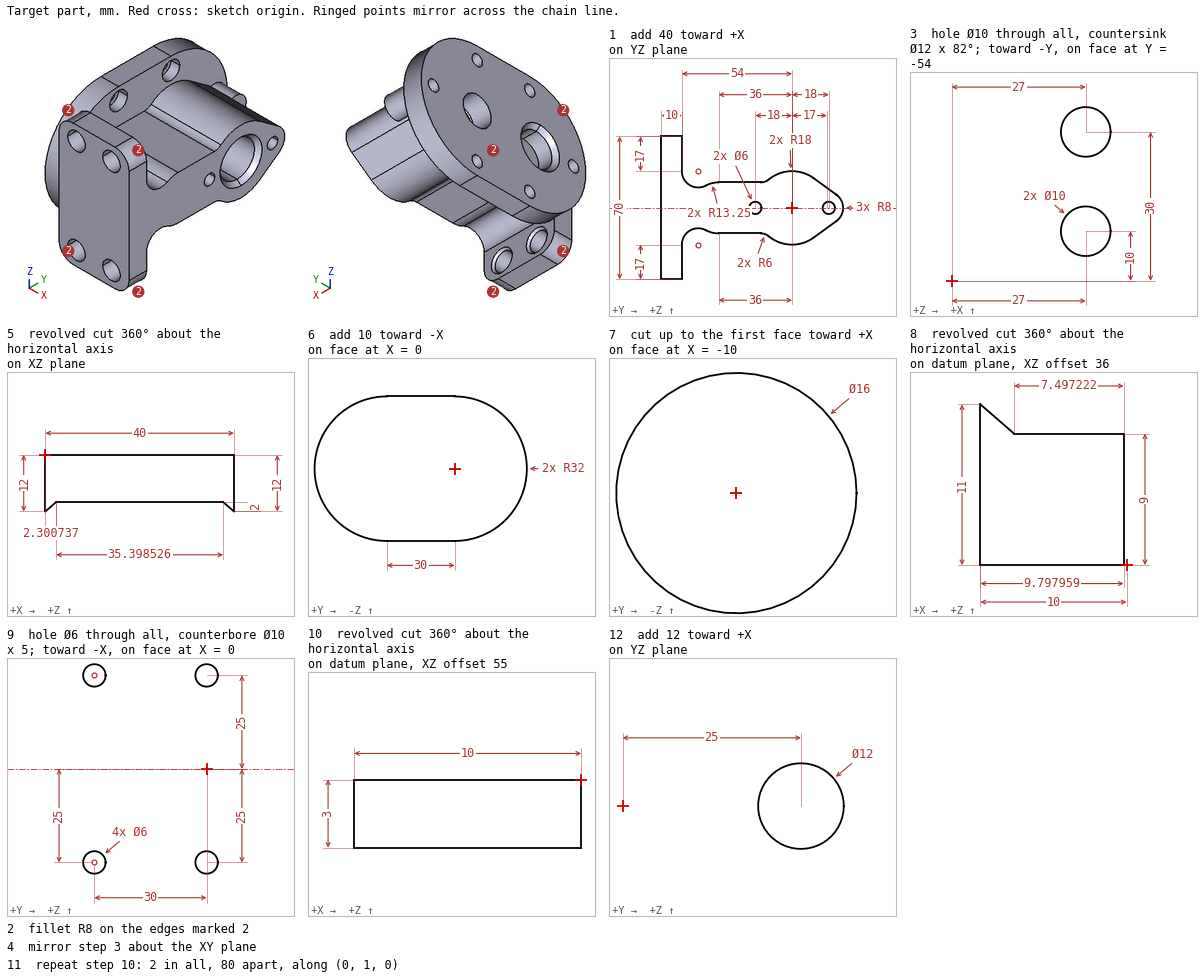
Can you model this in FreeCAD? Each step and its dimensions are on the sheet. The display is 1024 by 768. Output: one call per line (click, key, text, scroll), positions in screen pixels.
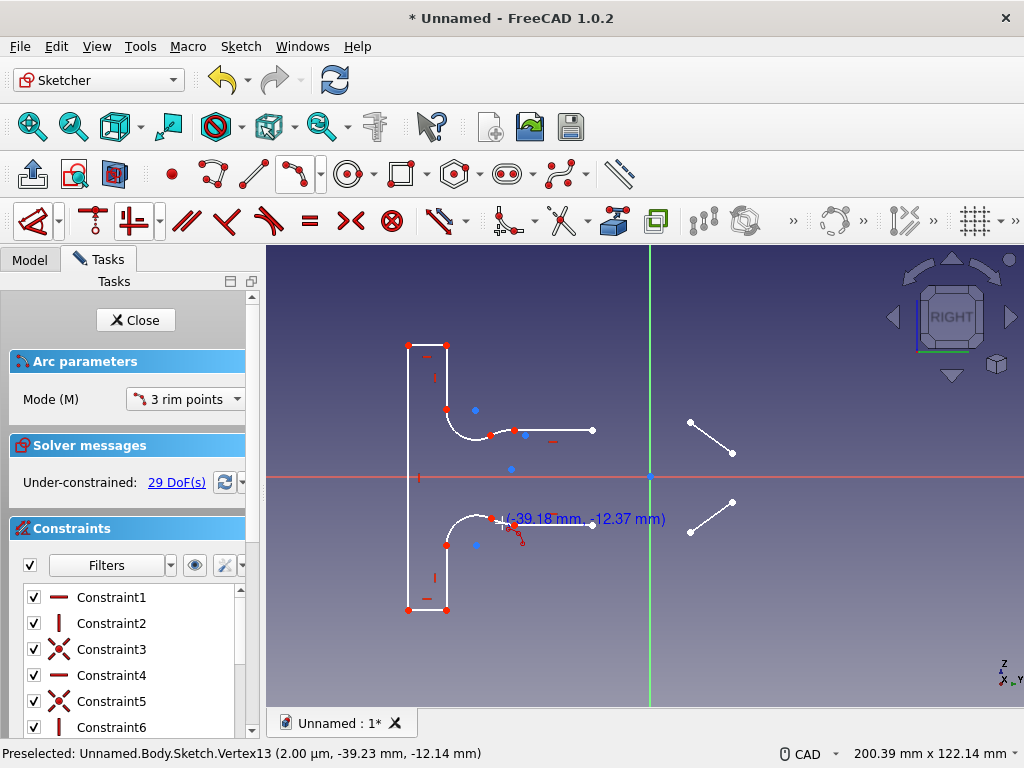
click(592, 525)
click(607, 529)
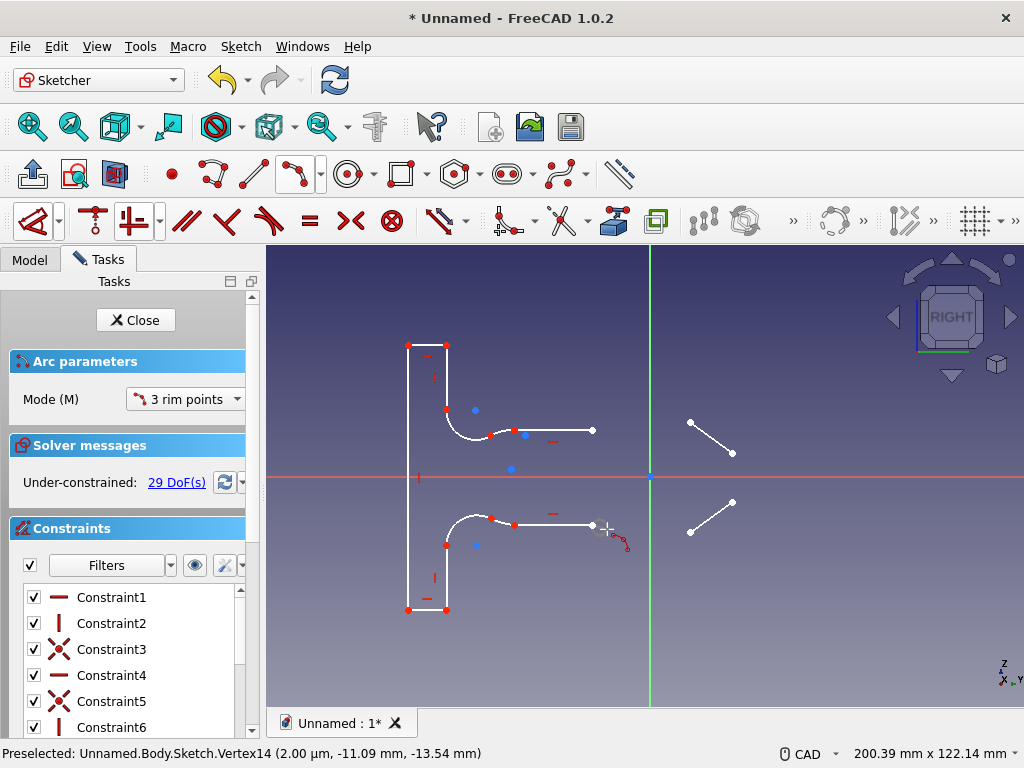
scroll(600, 525, up, 13)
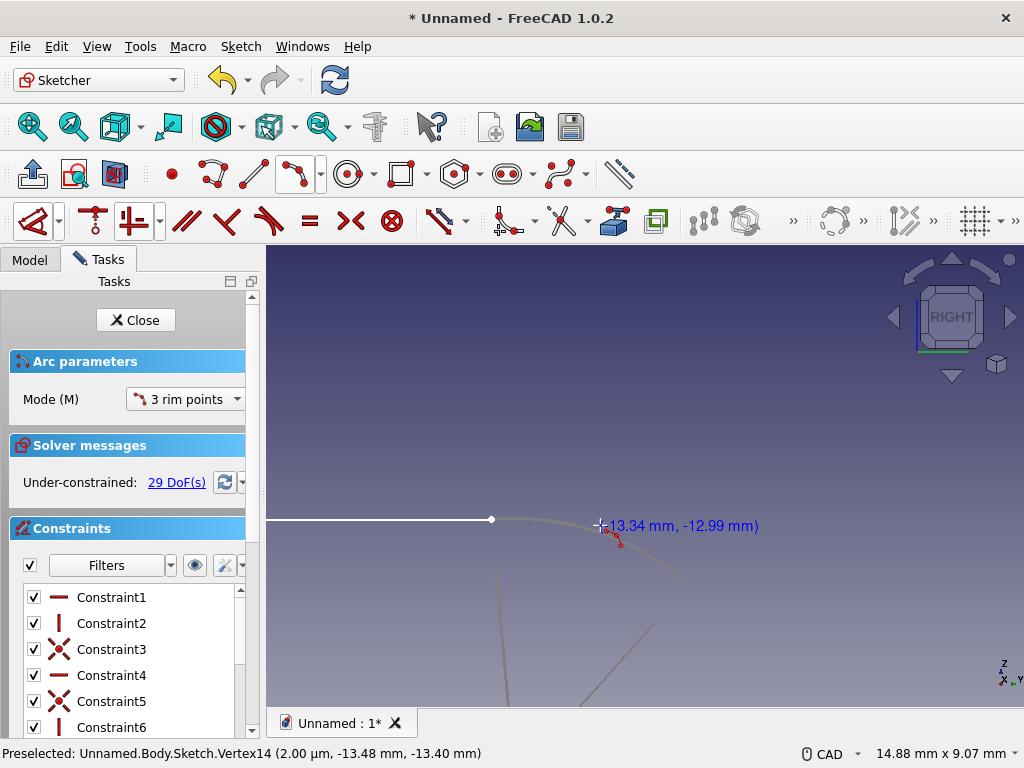
click(599, 524)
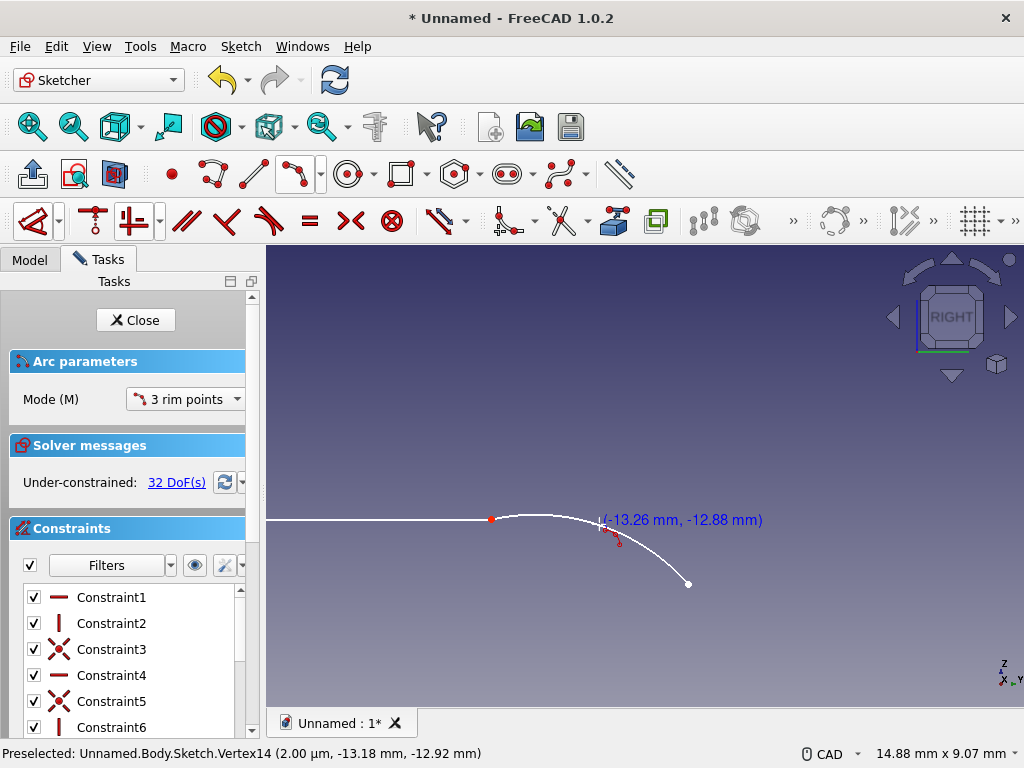
scroll(600, 525, down, 13)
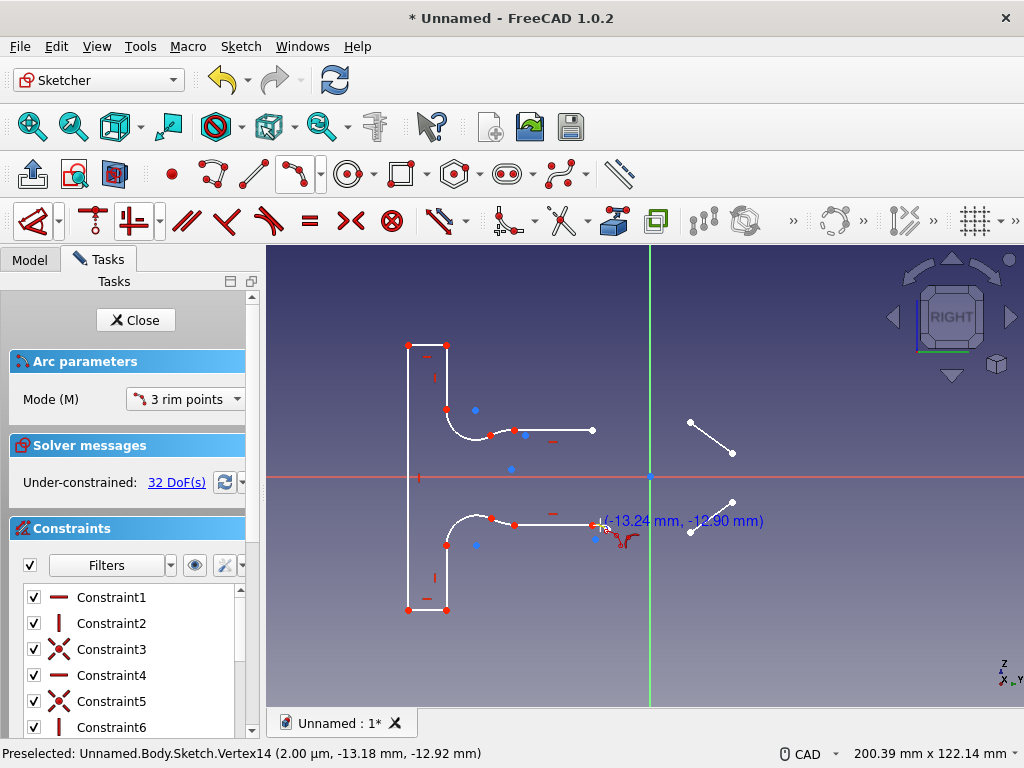
click(607, 530)
click(691, 533)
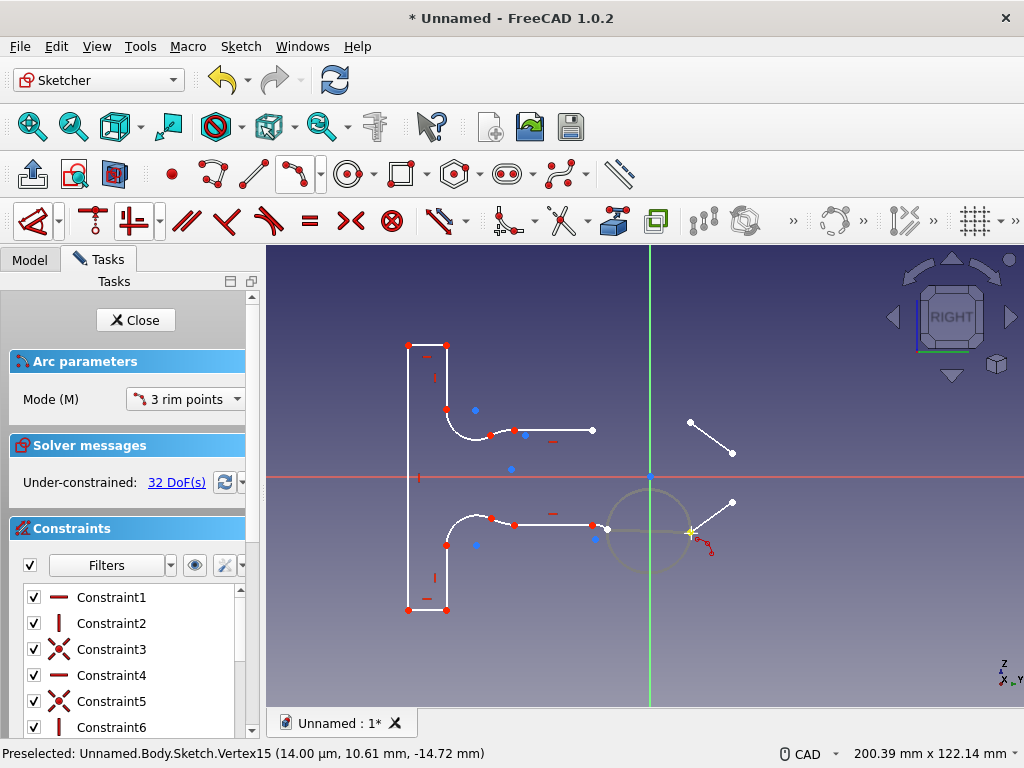
scroll(631, 542, up, 2)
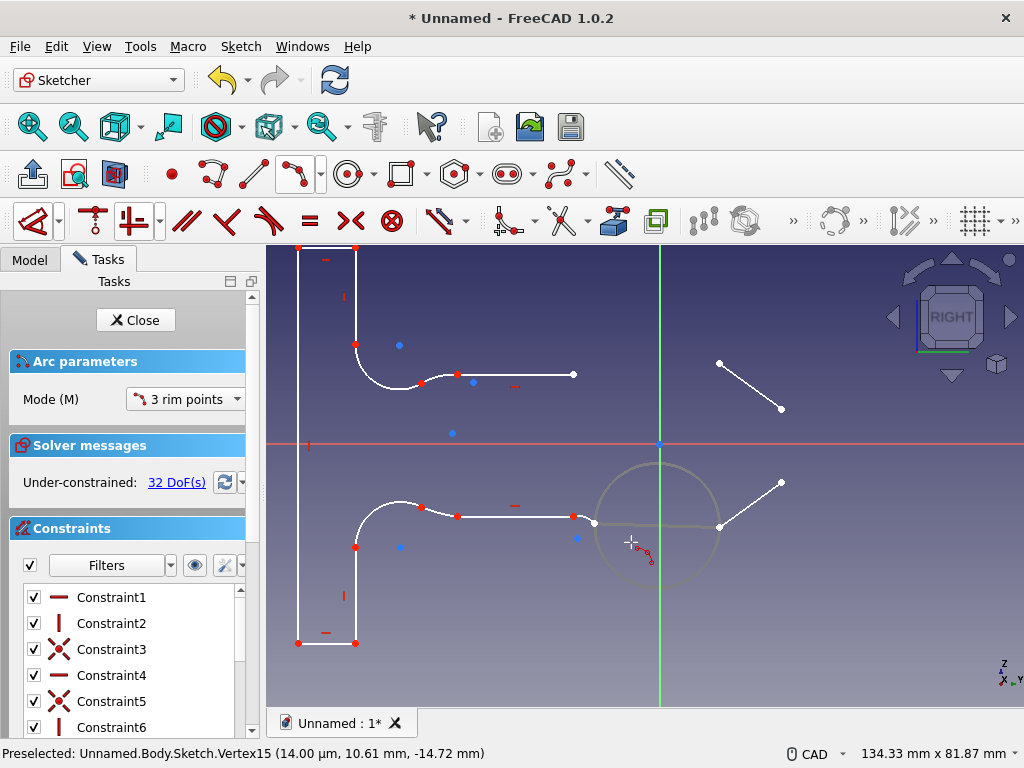
click(630, 542)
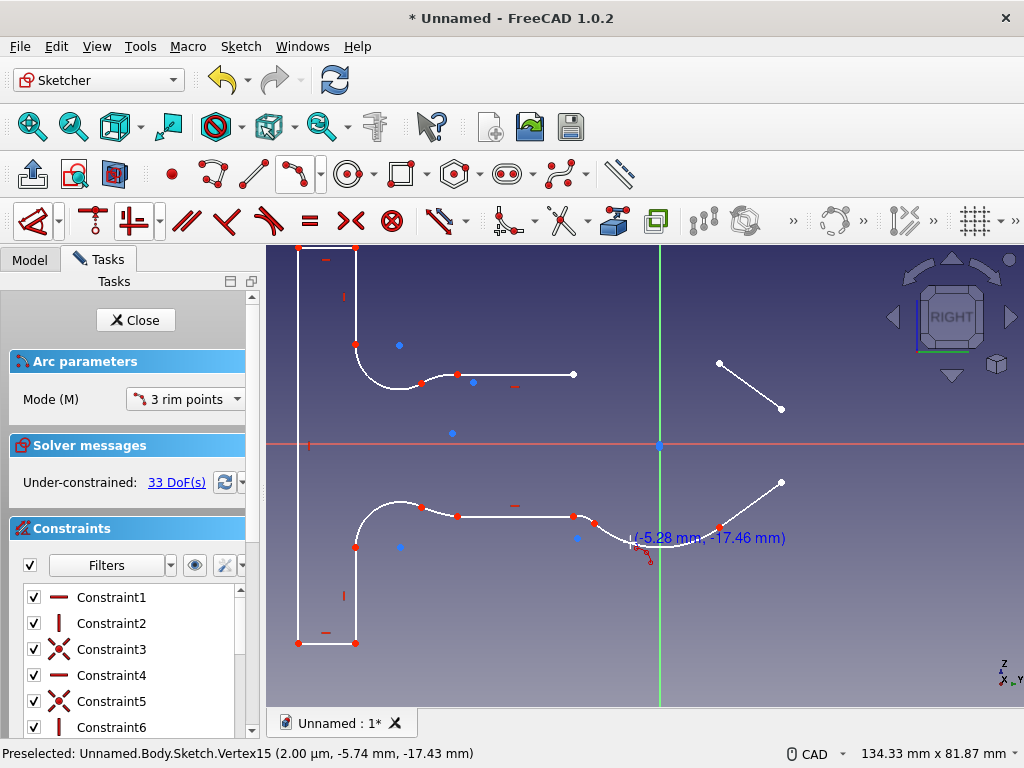
click(782, 482)
click(782, 409)
click(798, 461)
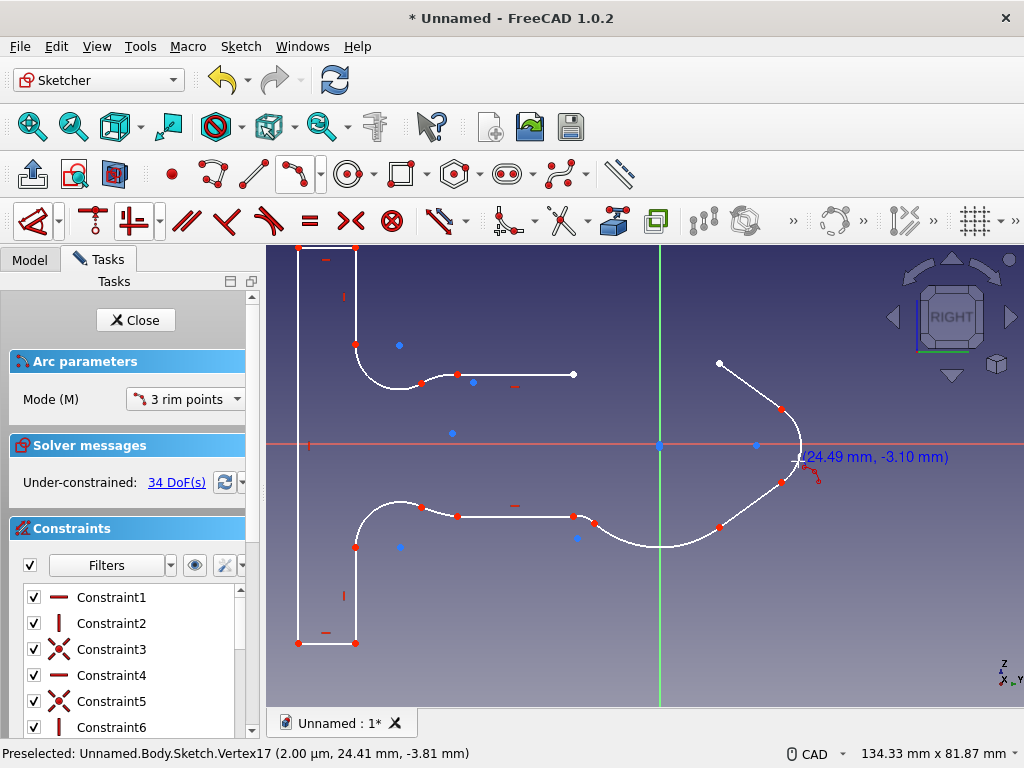
click(720, 364)
click(595, 366)
click(683, 346)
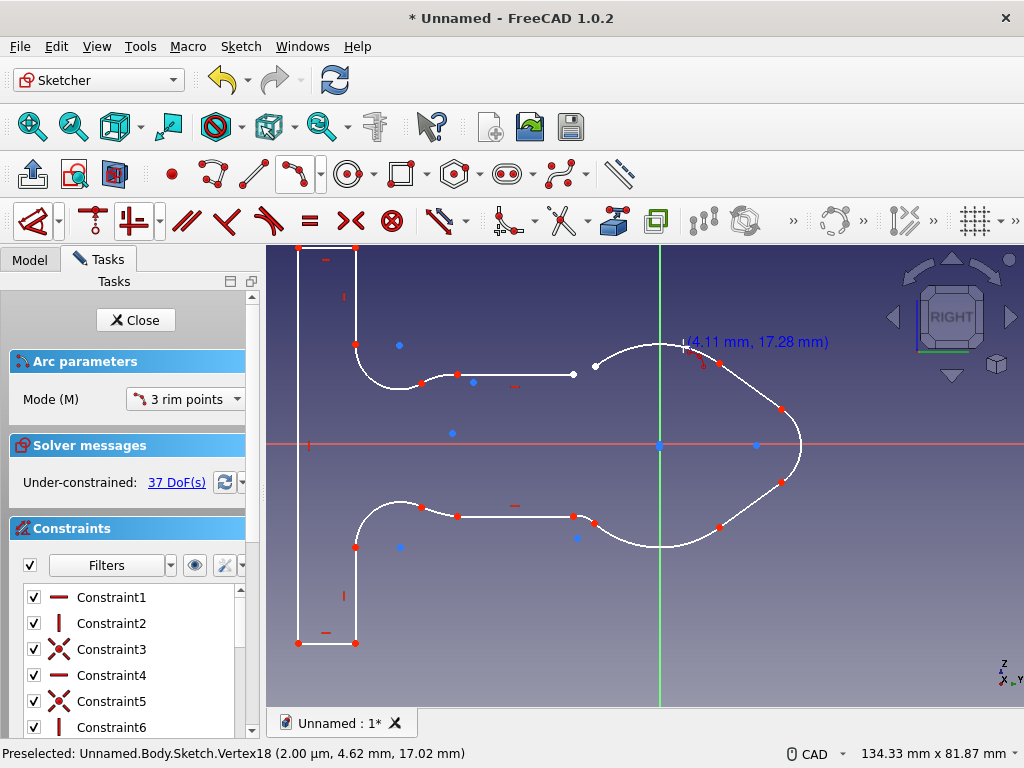
click(595, 367)
click(573, 375)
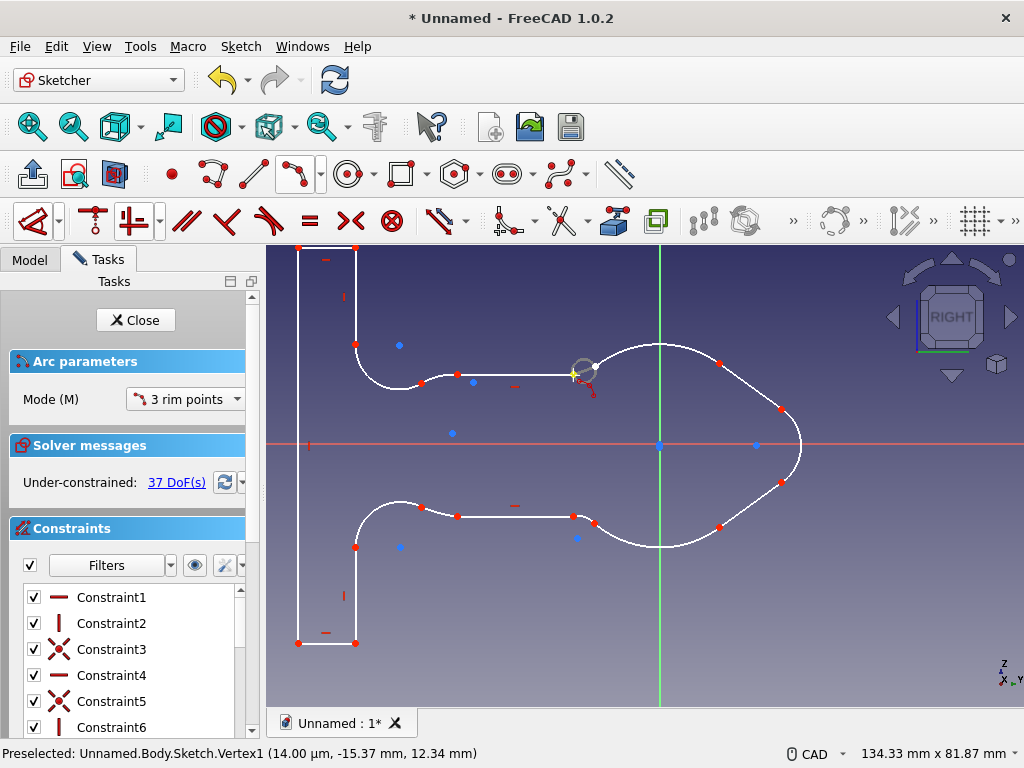
scroll(585, 372, up, 11)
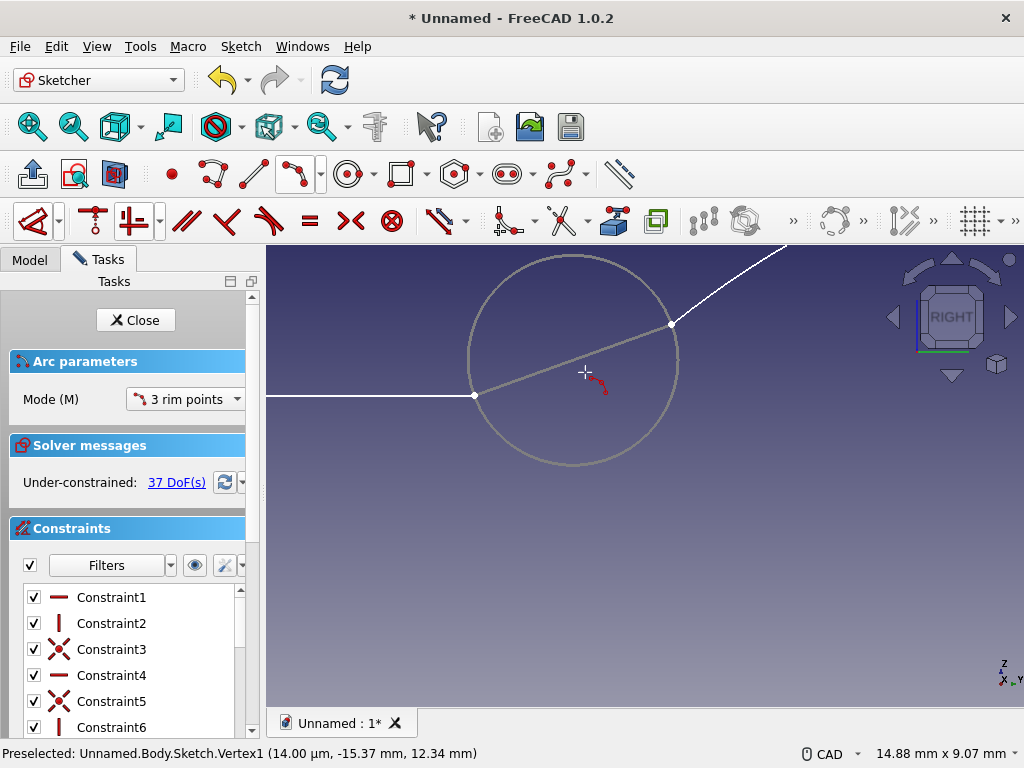
click(582, 369)